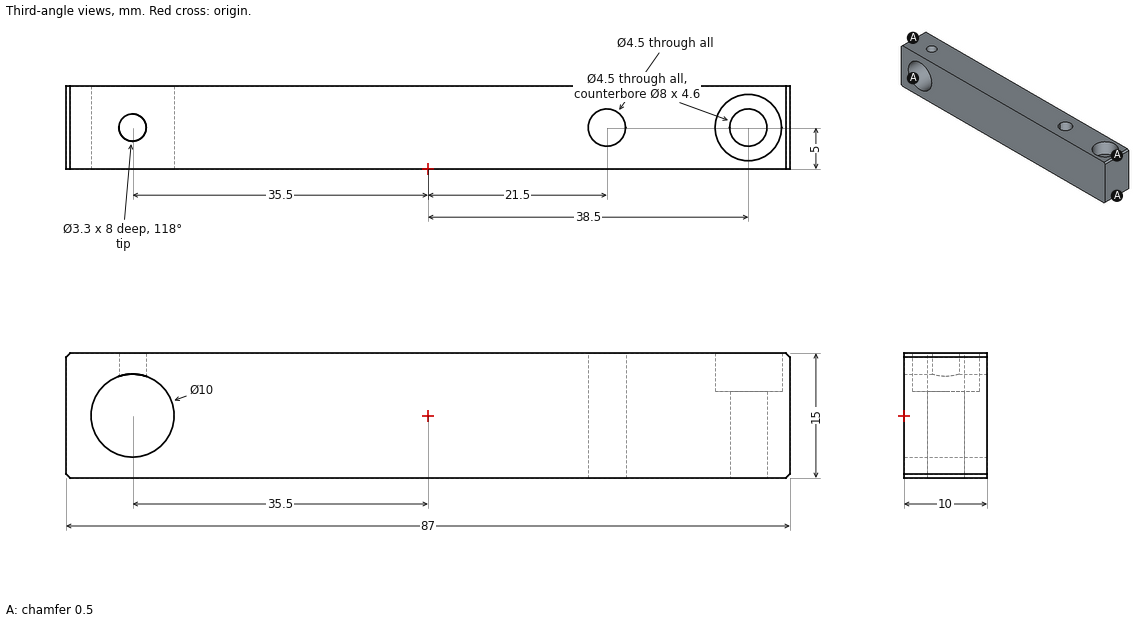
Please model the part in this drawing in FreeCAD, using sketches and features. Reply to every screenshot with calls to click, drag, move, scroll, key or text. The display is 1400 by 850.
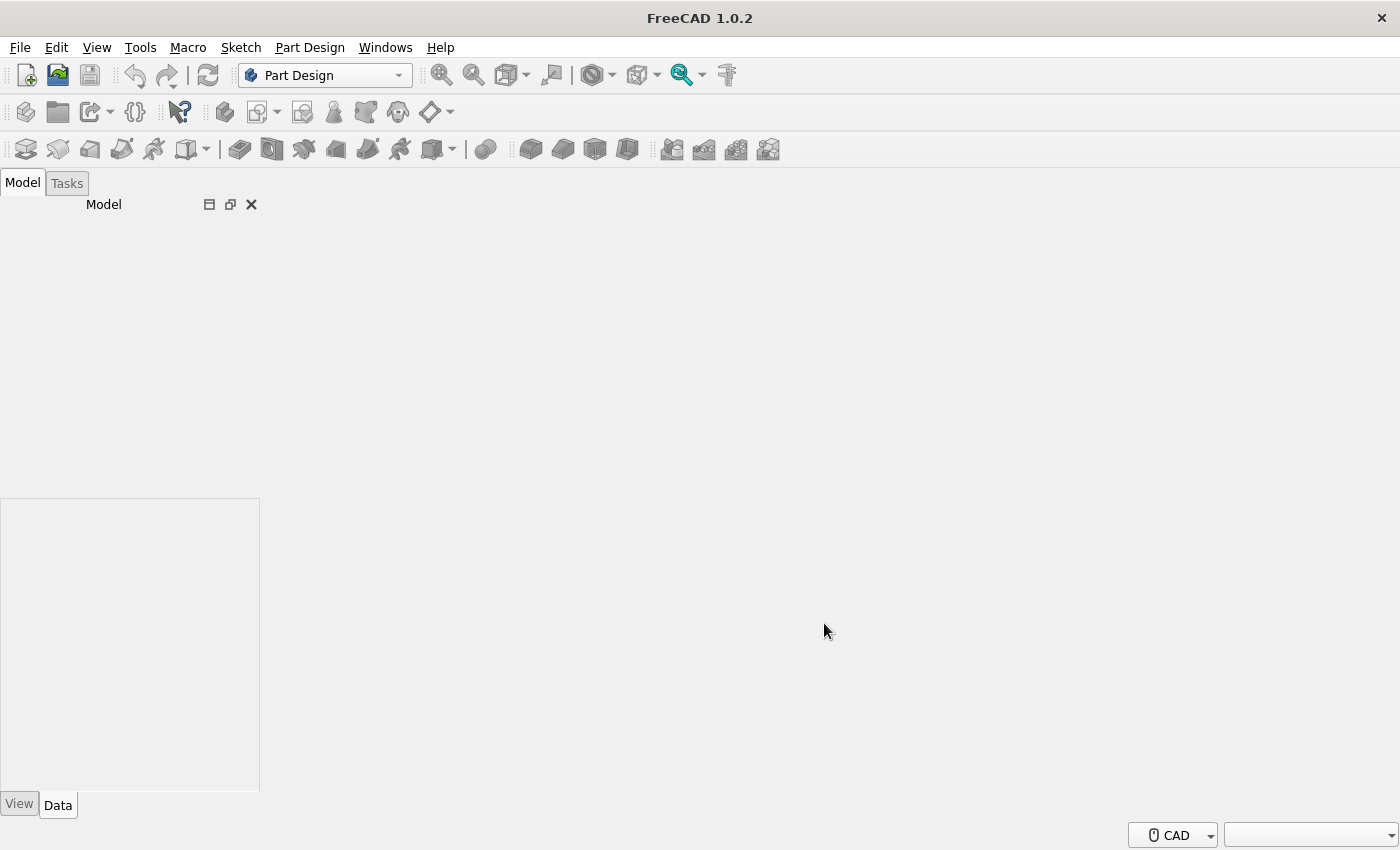
click(26, 76)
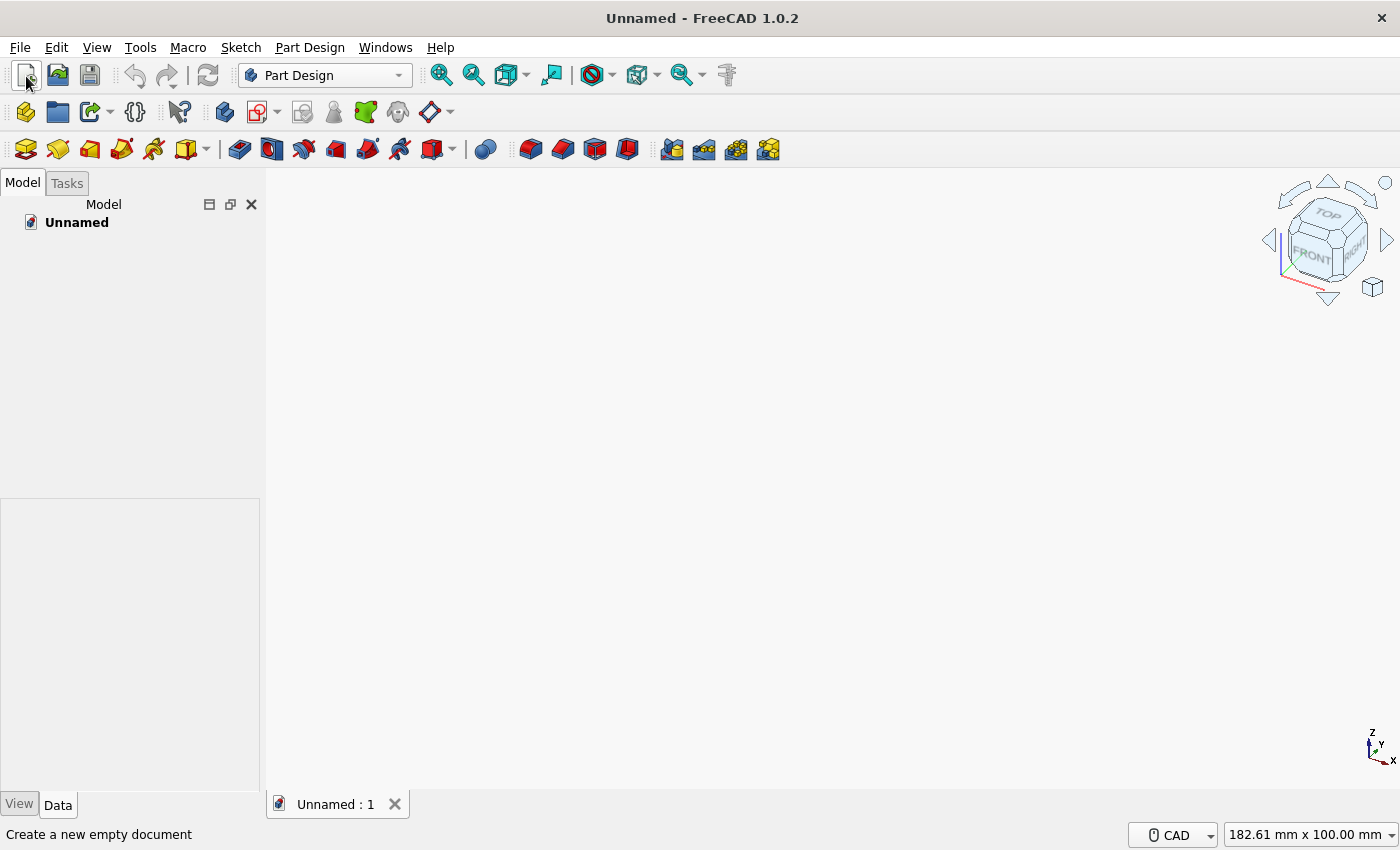
click(258, 112)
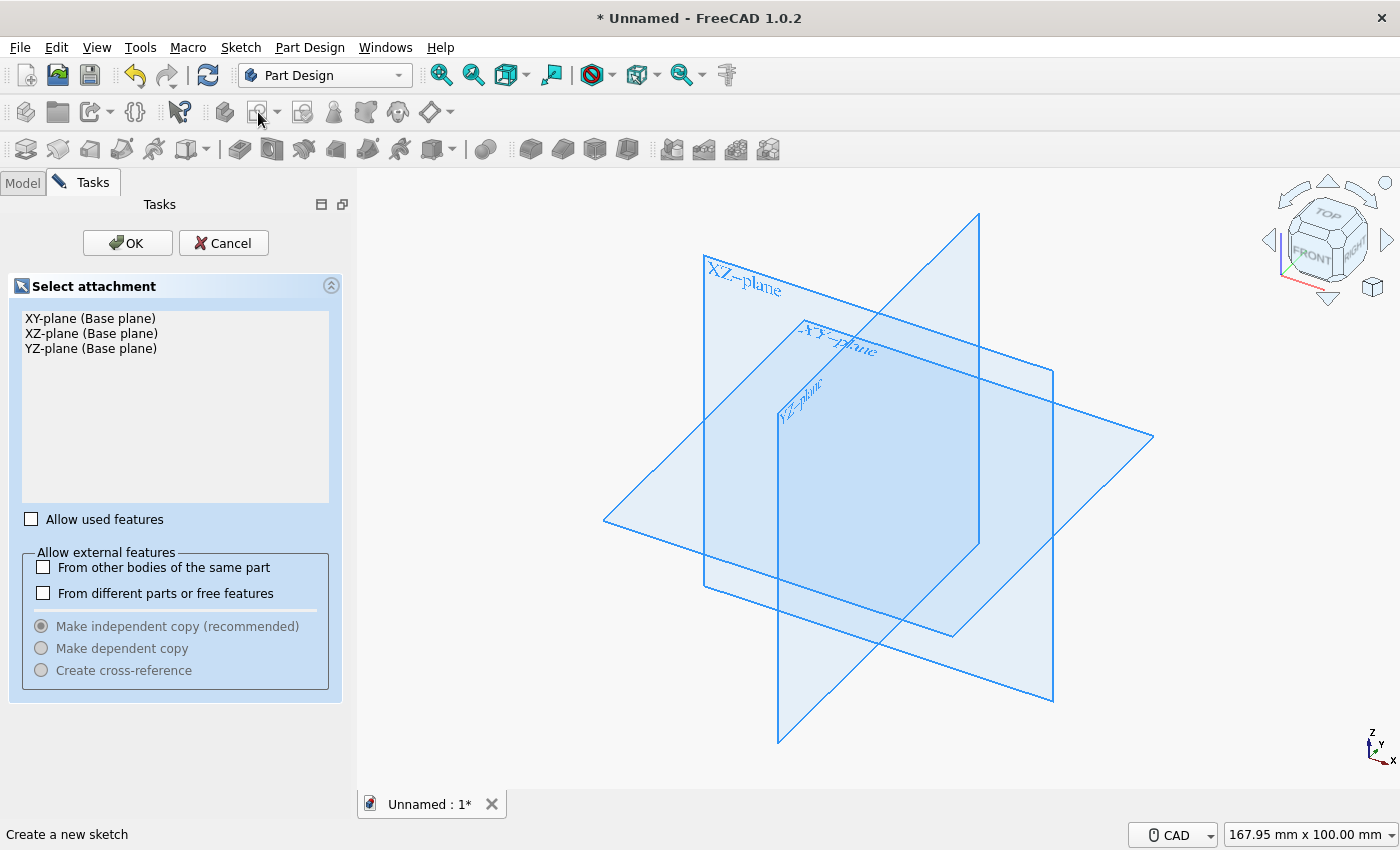
click(82, 334)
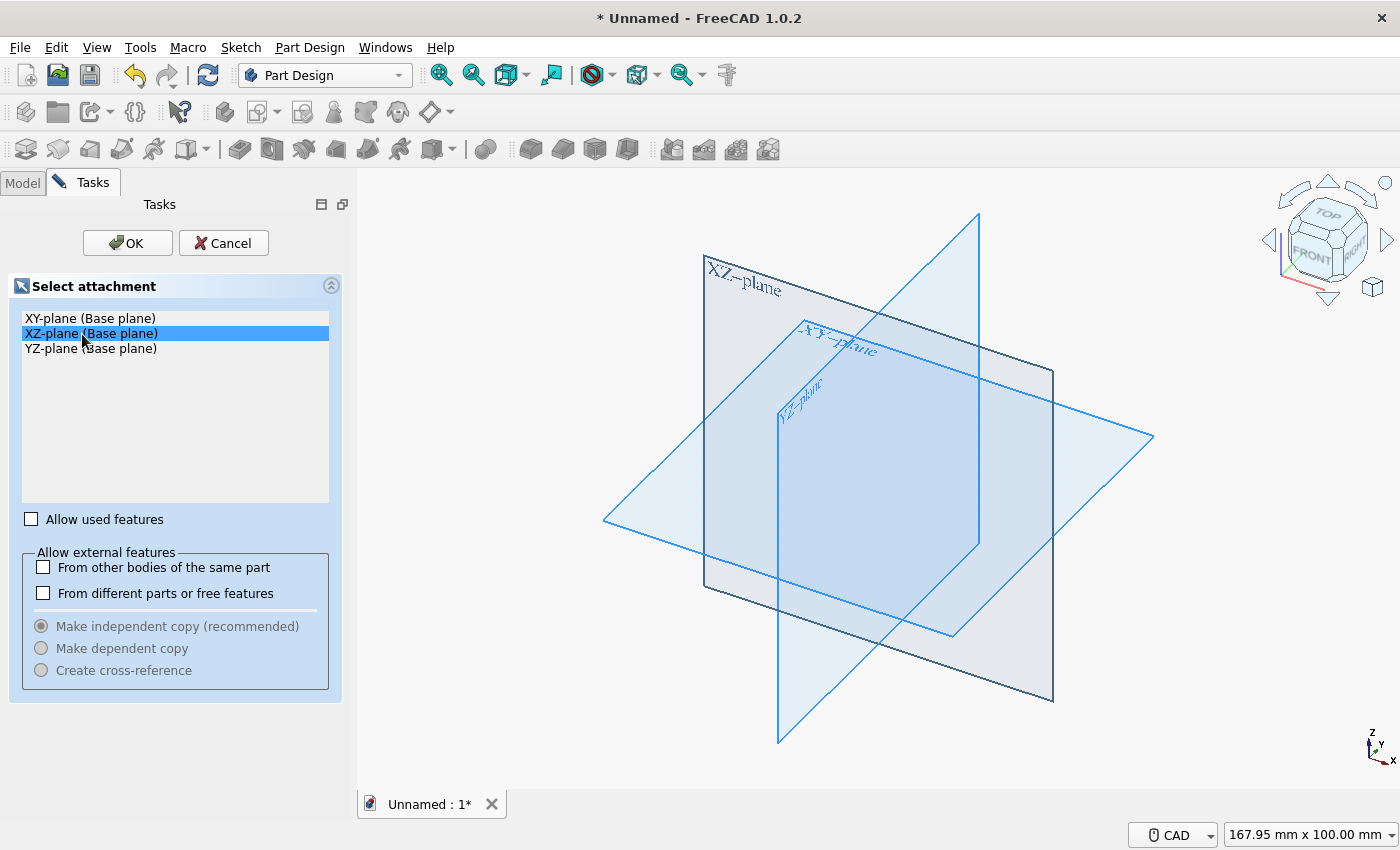
click(128, 243)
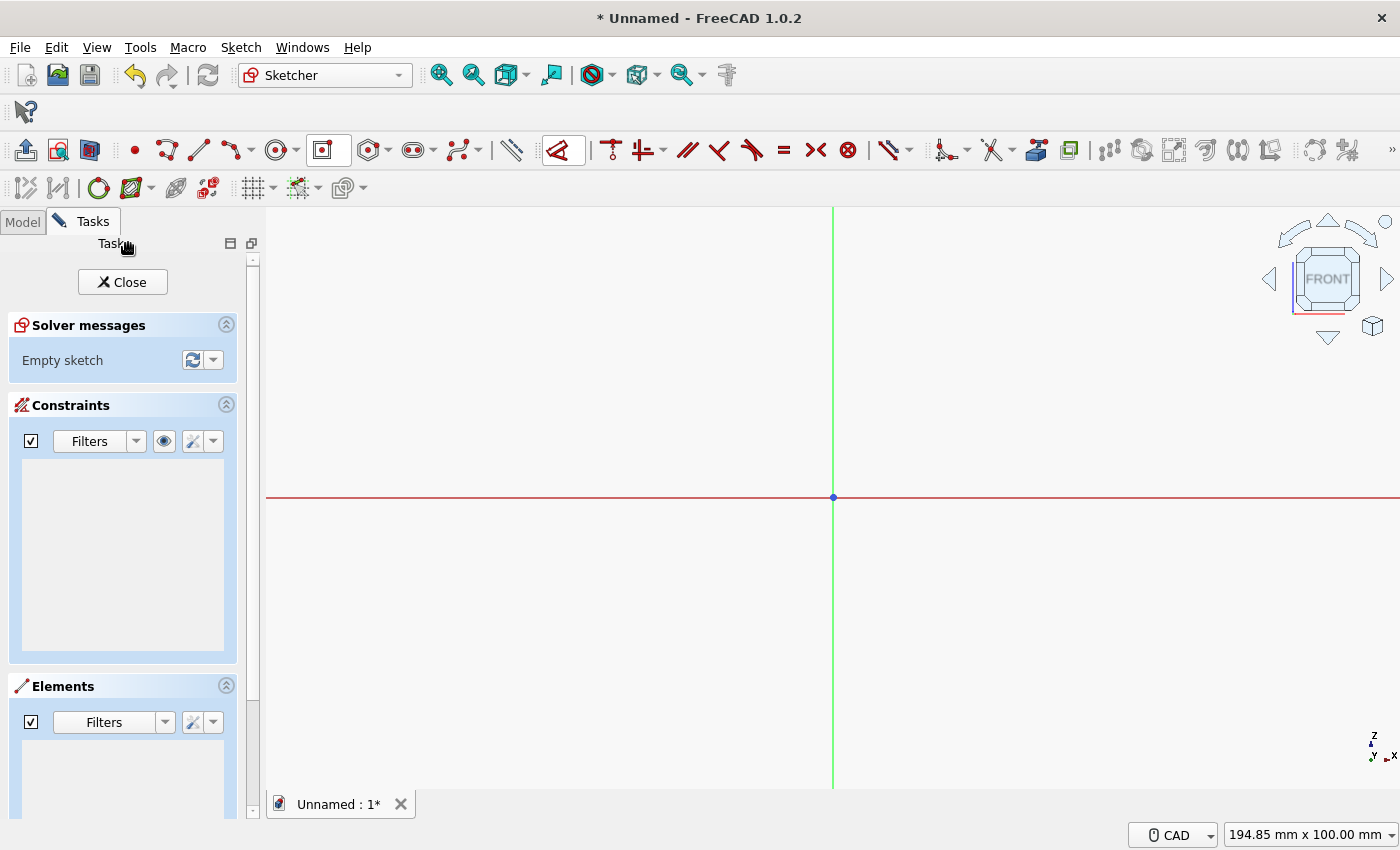
click(322, 150)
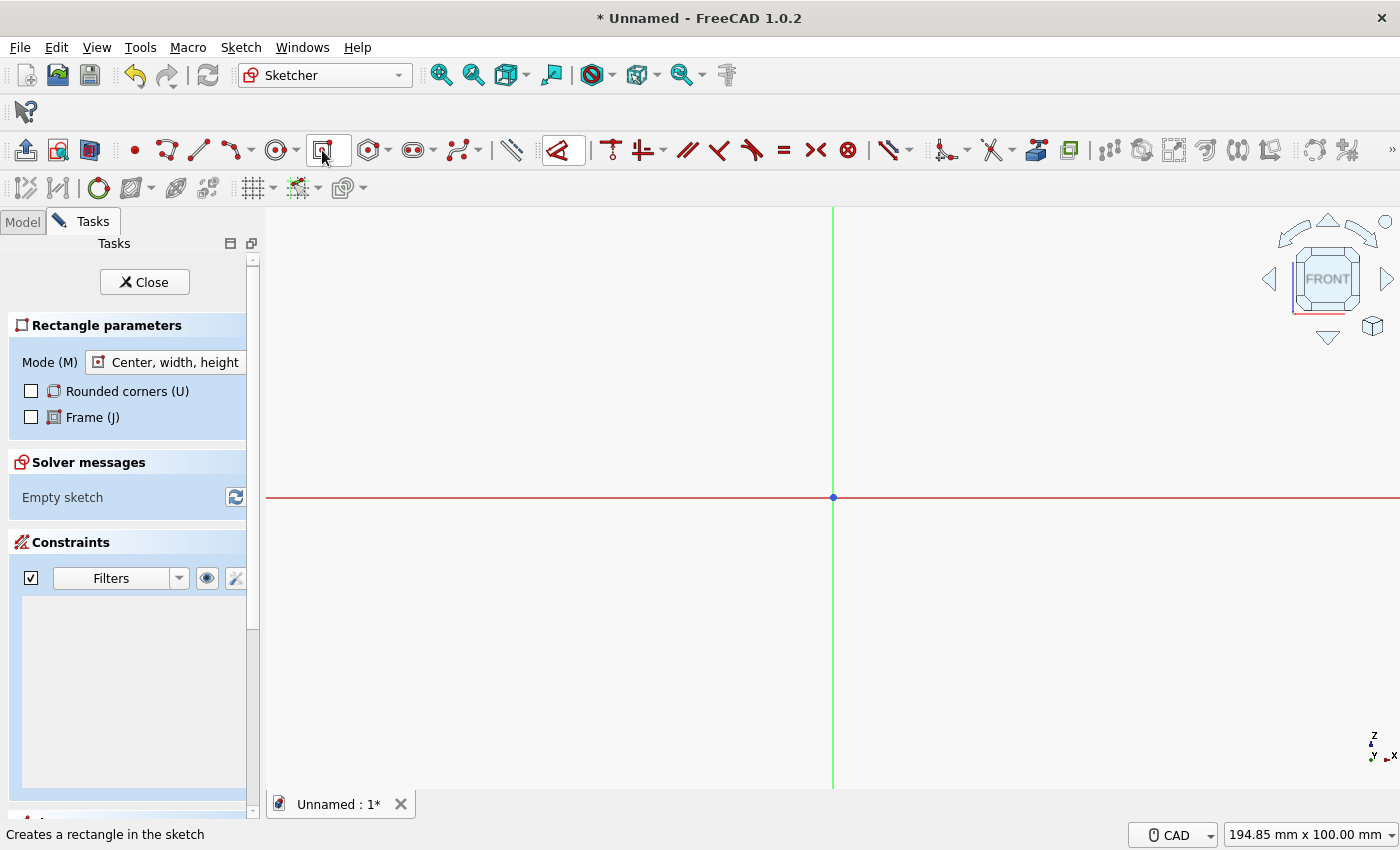
click(833, 498)
click(1086, 454)
key(Escape)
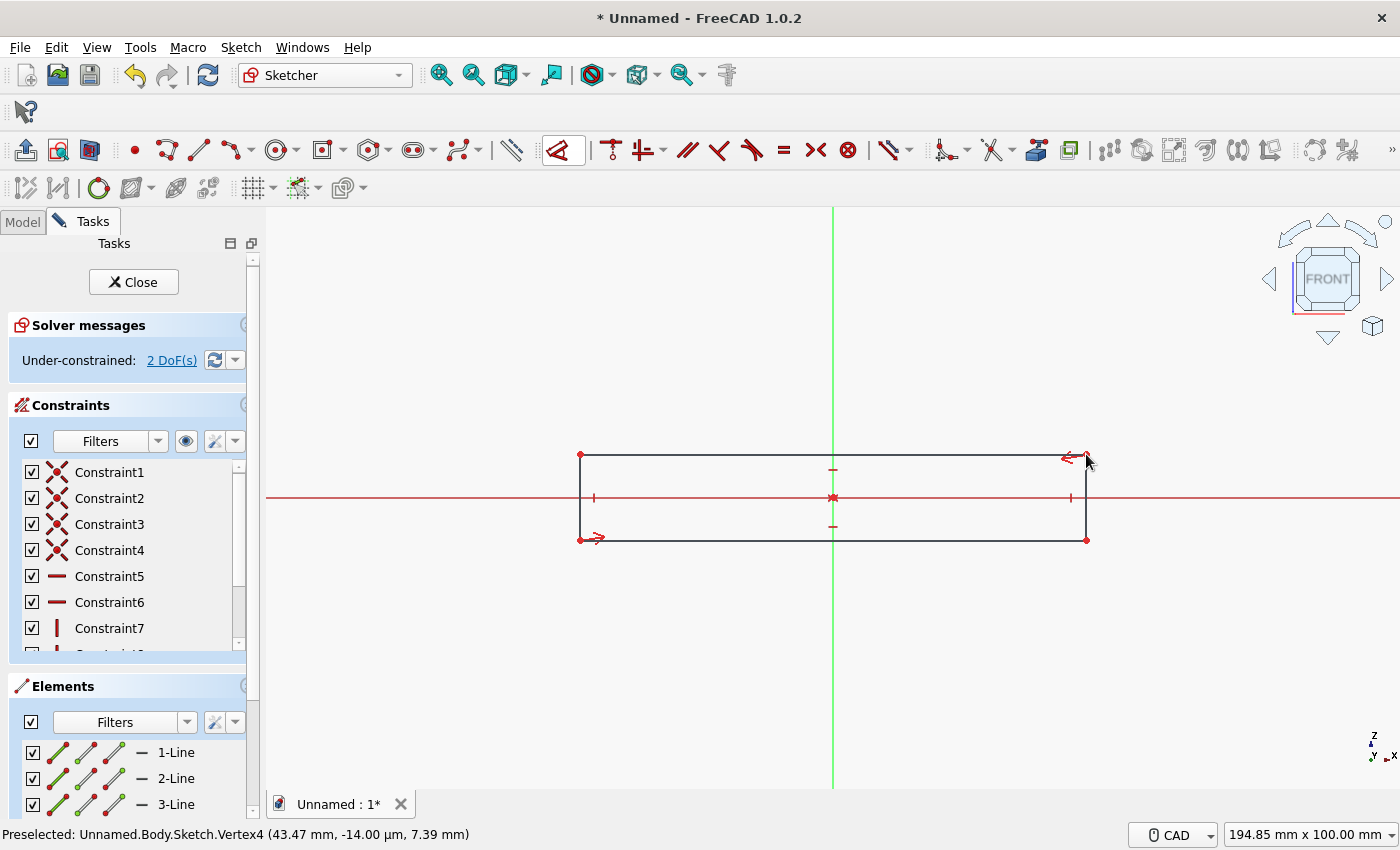
click(558, 150)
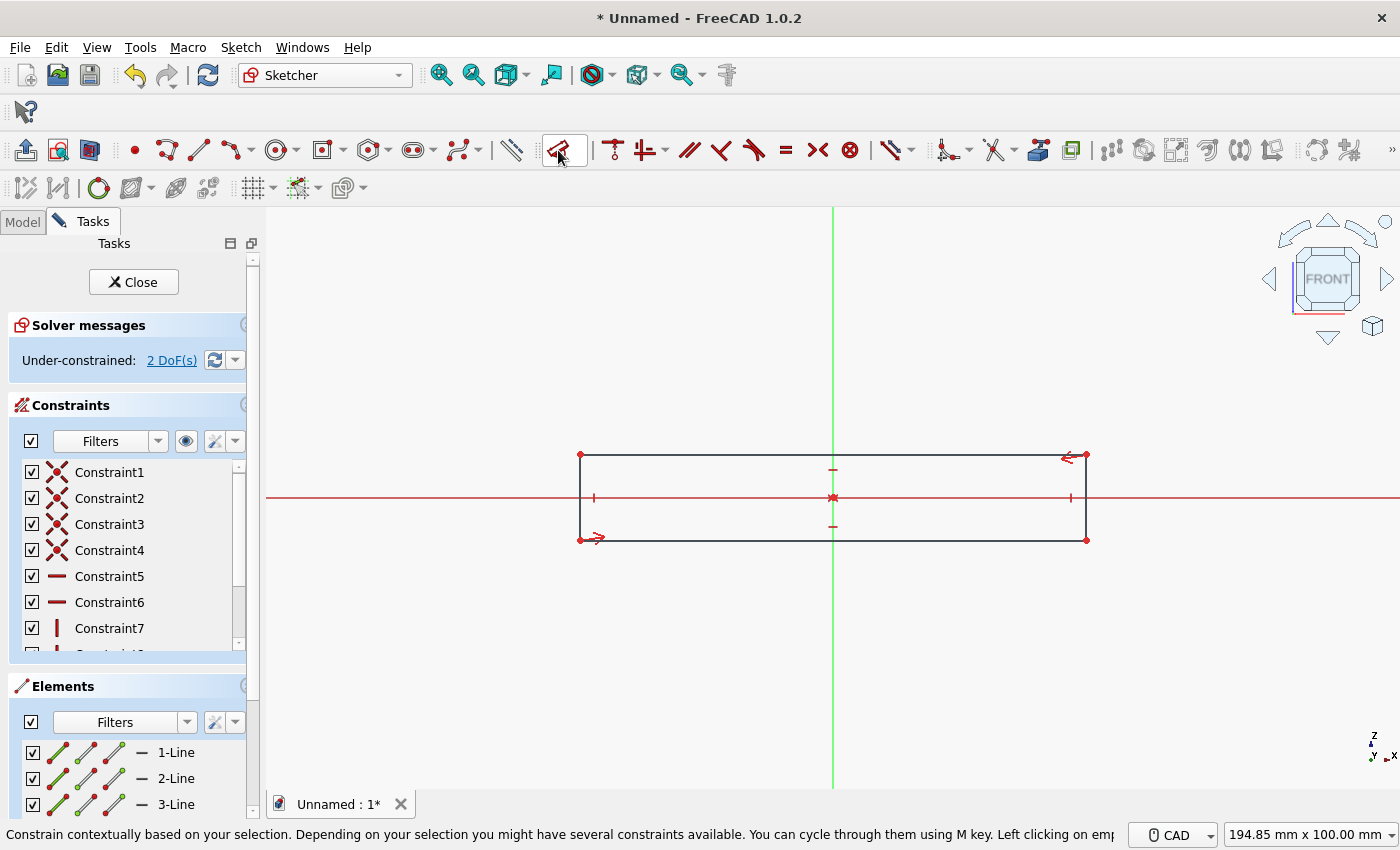
click(732, 541)
click(717, 575)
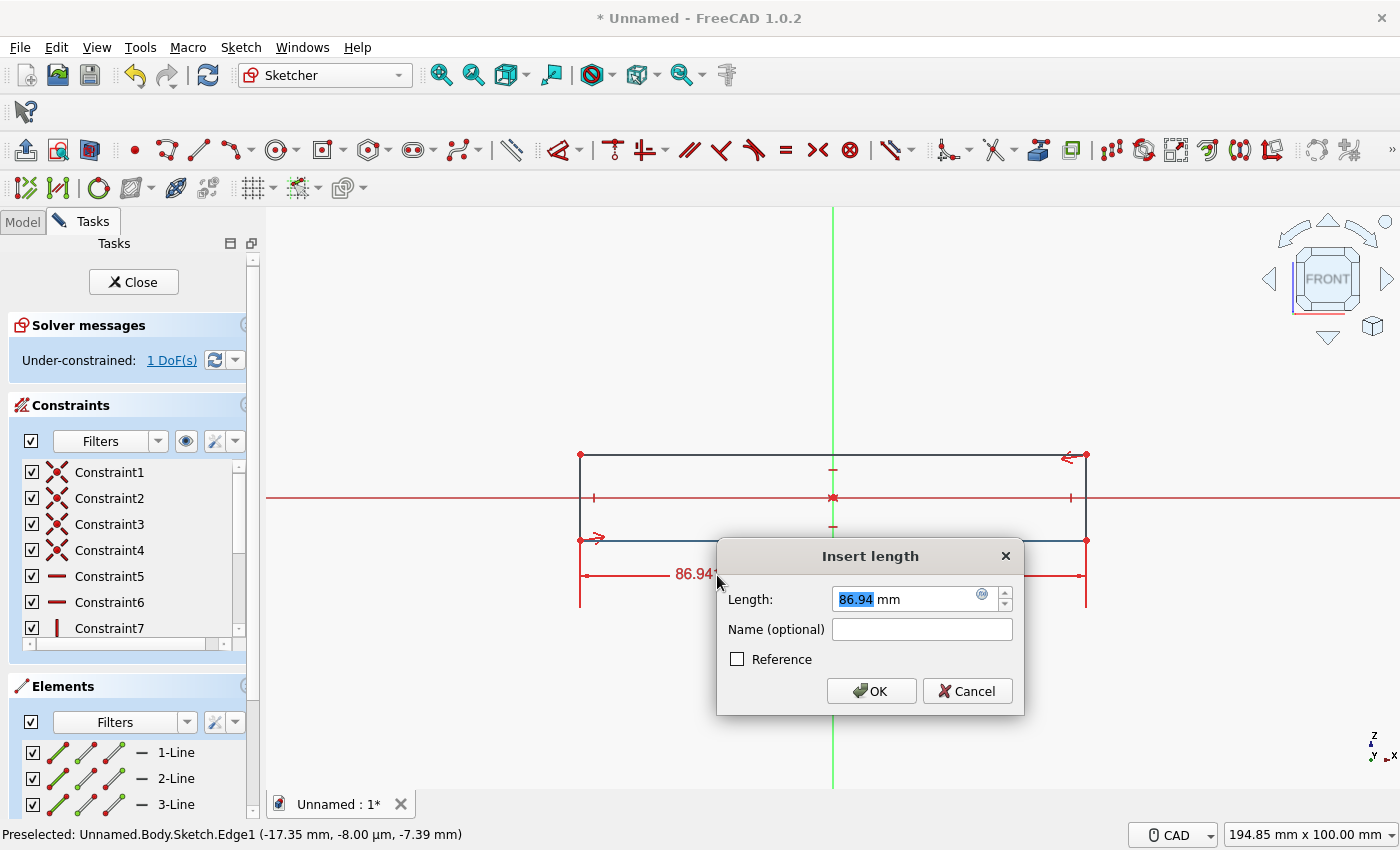
text(87)
key(Return)